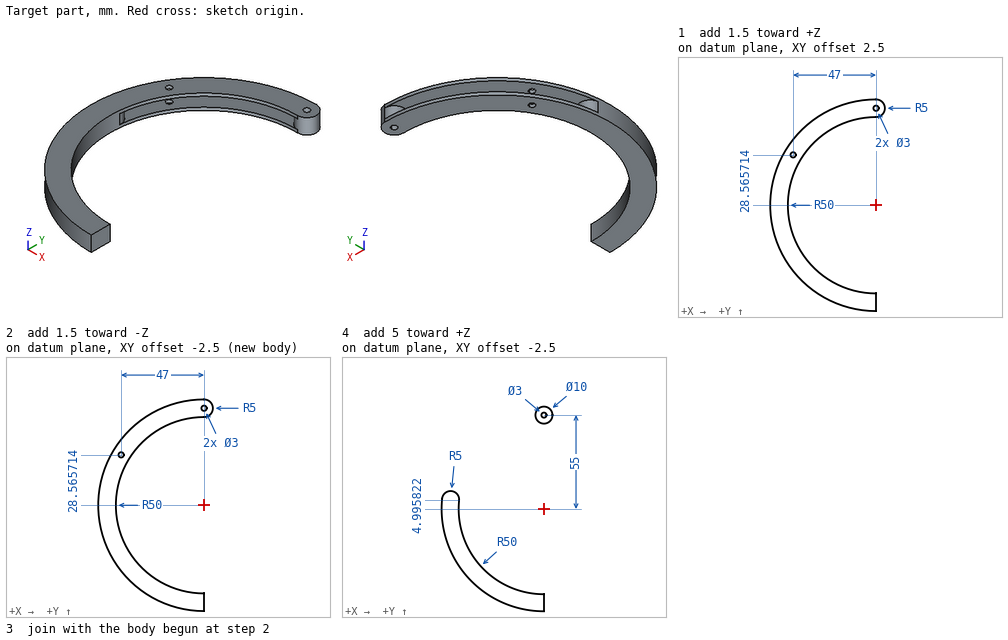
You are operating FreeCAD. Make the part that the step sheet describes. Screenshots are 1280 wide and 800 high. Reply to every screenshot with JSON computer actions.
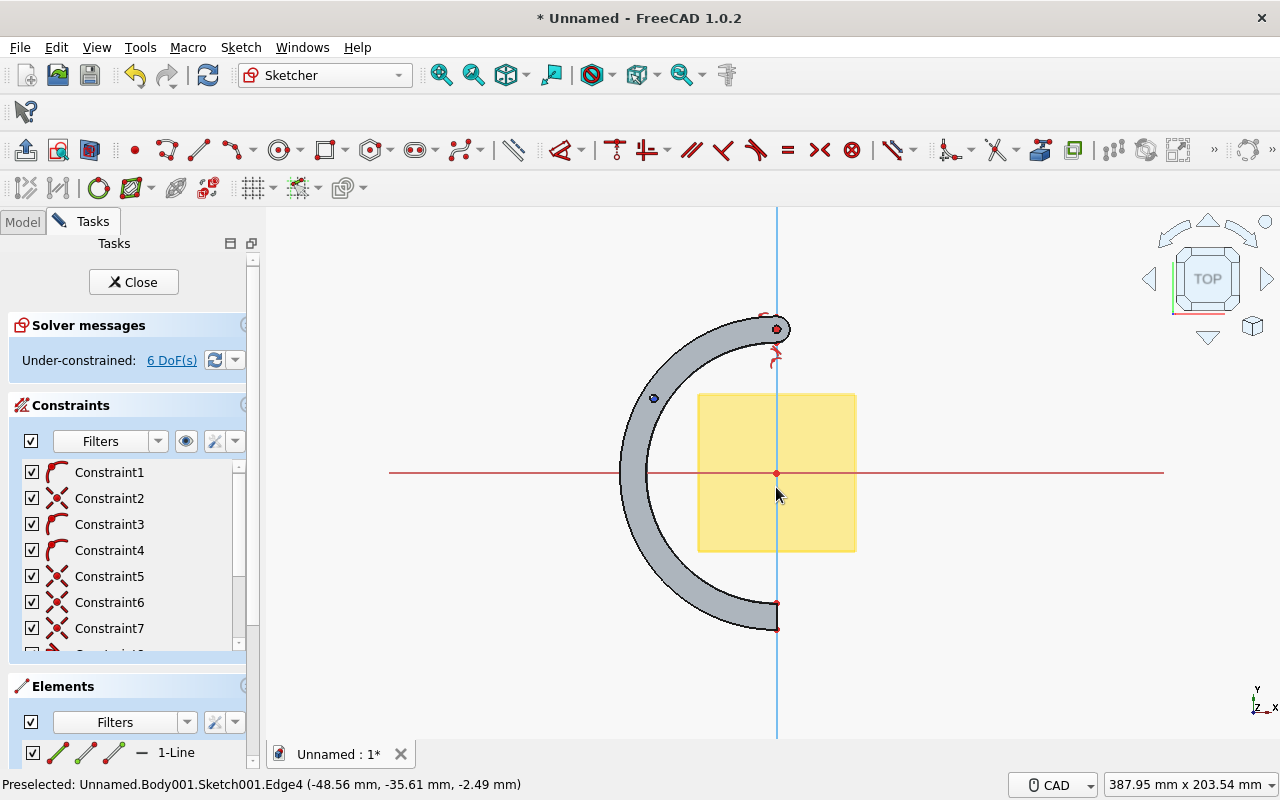
{"action": "scroll", "coordinate": [656, 398], "scroll_direction": "up", "scroll_amount": 8}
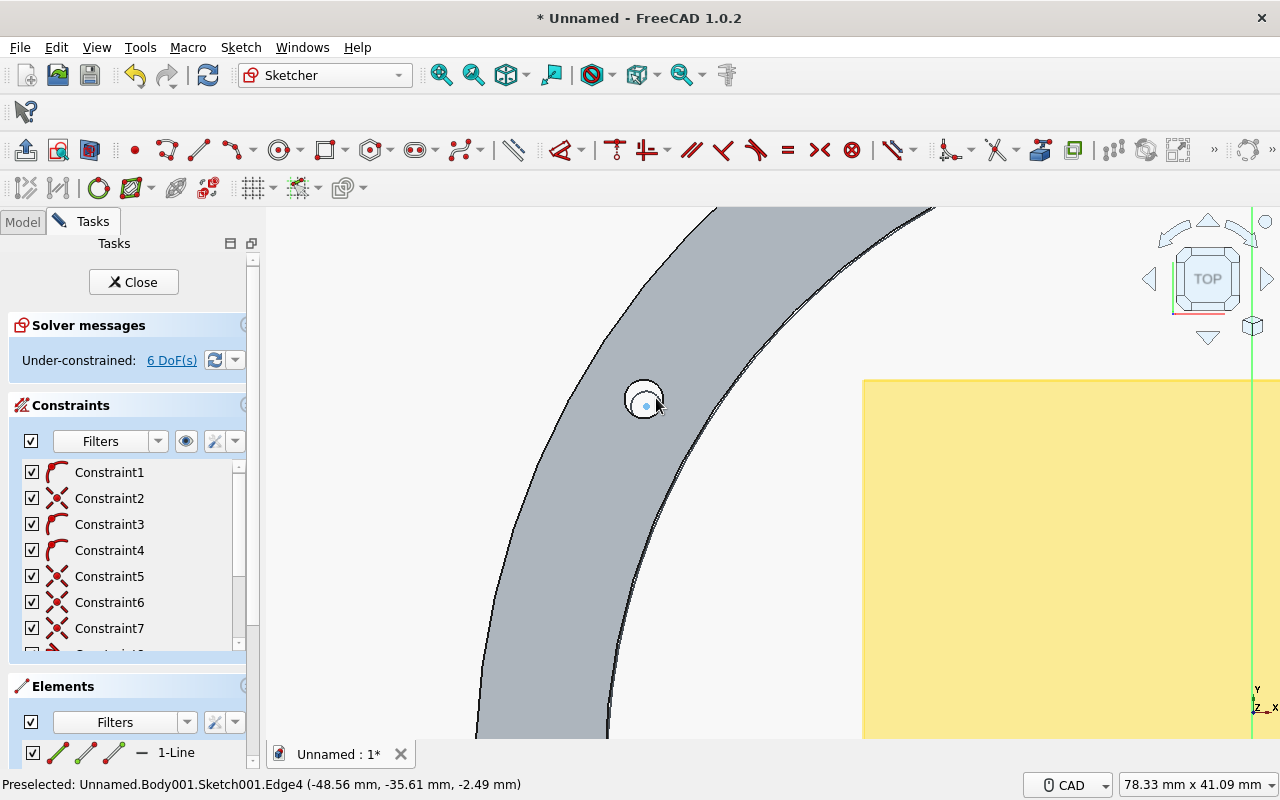
{"action": "left_click", "coordinate": [657, 396]}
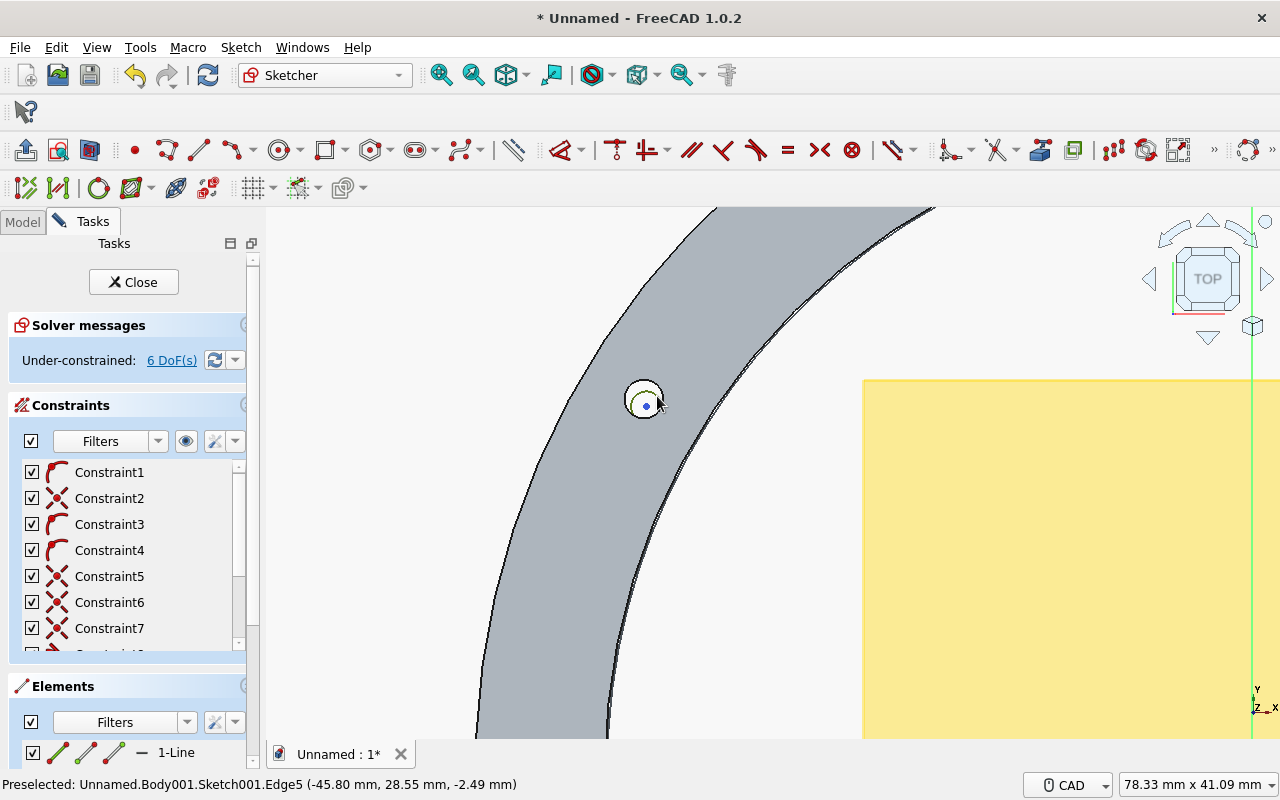
{"action": "scroll", "coordinate": [656, 398], "scroll_direction": "down", "scroll_amount": 8}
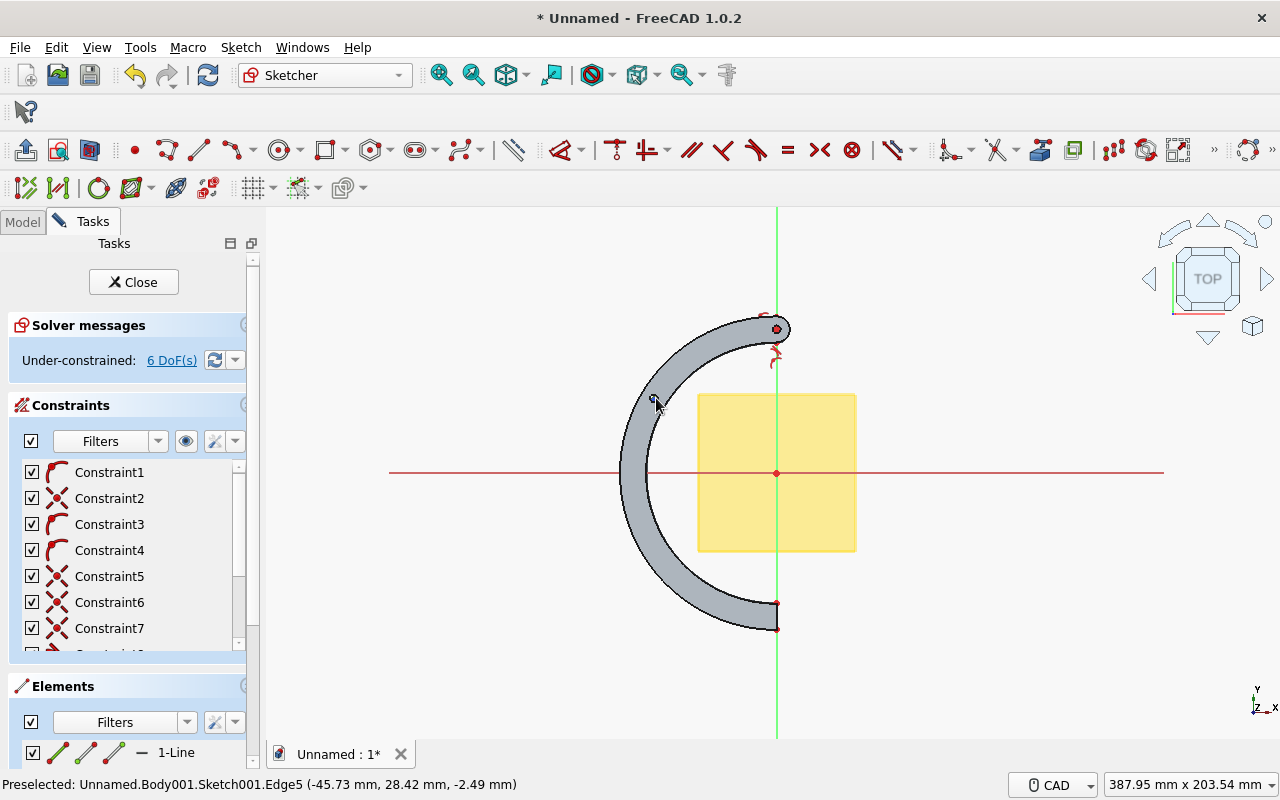
{"action": "scroll", "coordinate": [780, 327], "scroll_direction": "up", "scroll_amount": 8}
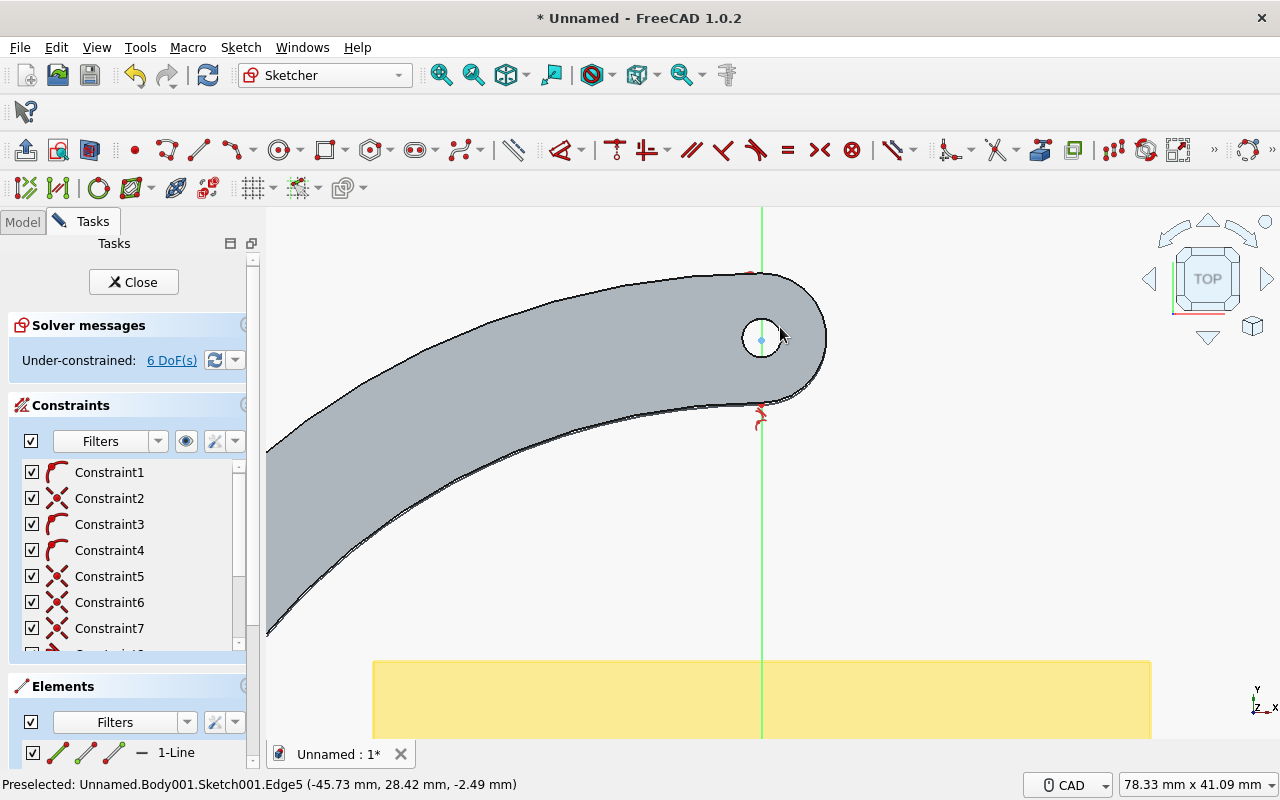
{"action": "left_click", "coordinate": [777, 325]}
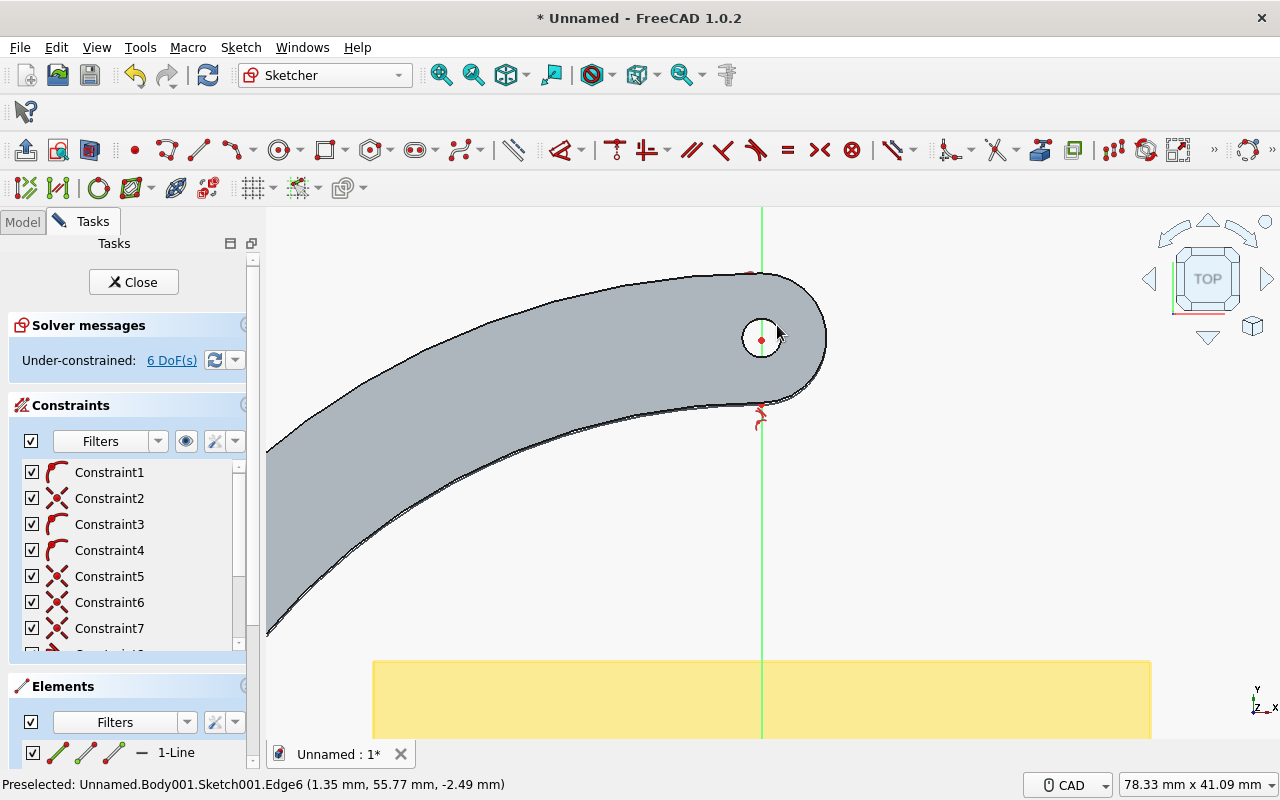
{"action": "left_click", "coordinate": [788, 150]}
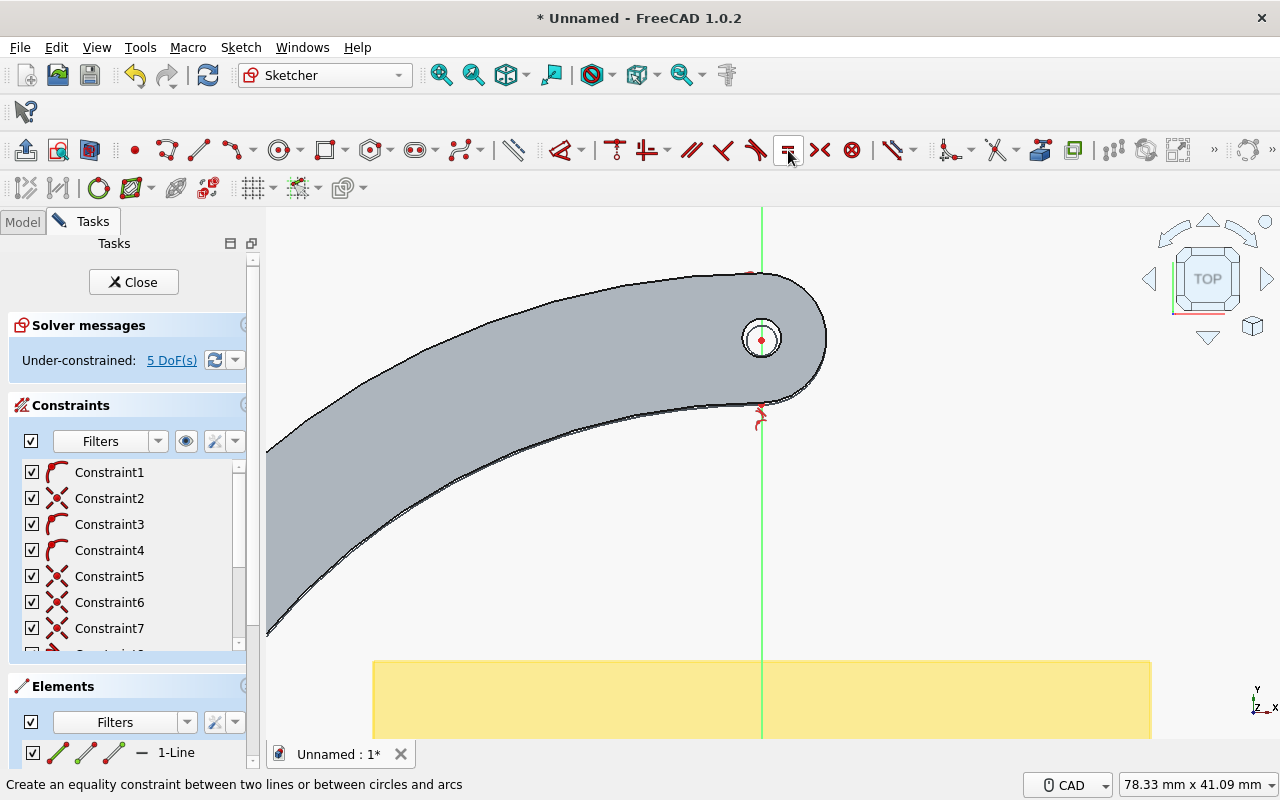
{"action": "left_click", "coordinate": [560, 150]}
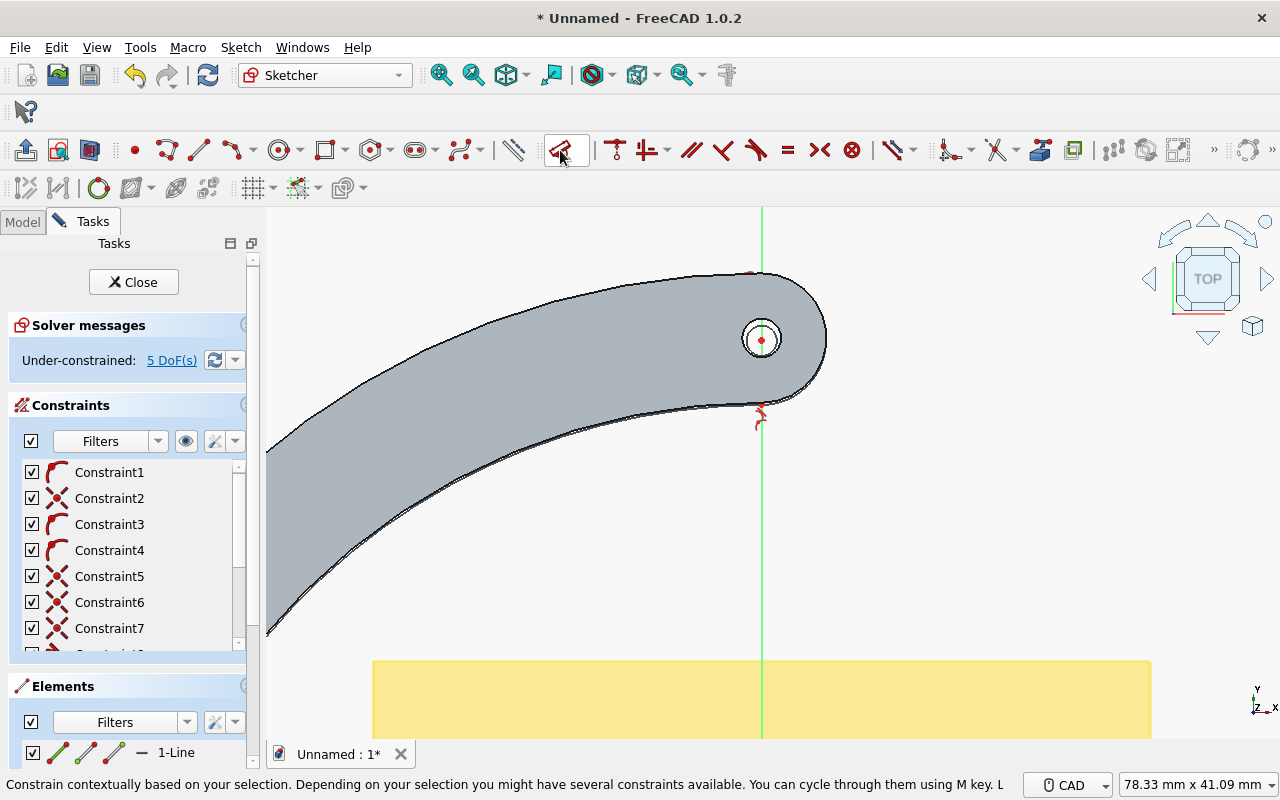
{"action": "scroll", "coordinate": [780, 327], "scroll_direction": "down", "scroll_amount": 8}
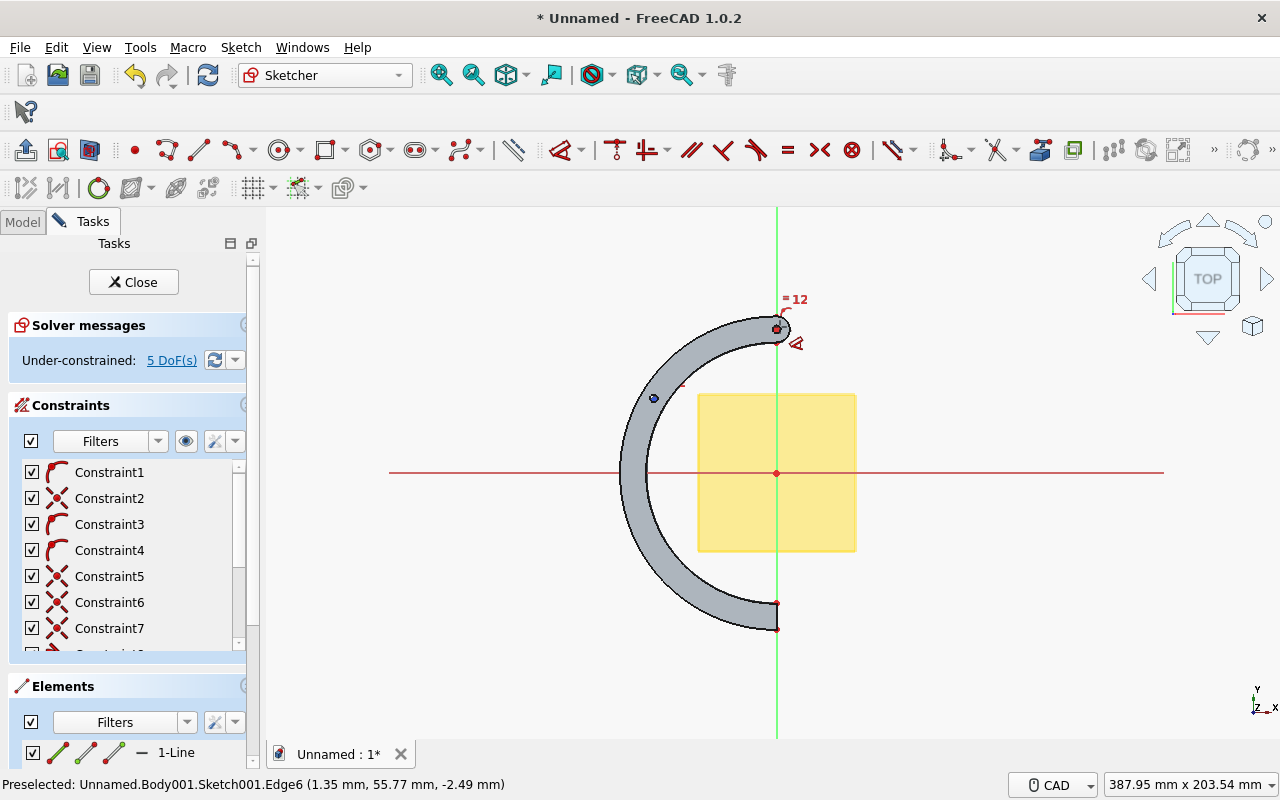
{"action": "left_click", "coordinate": [700, 368]}
{"action": "left_click", "coordinate": [835, 322]}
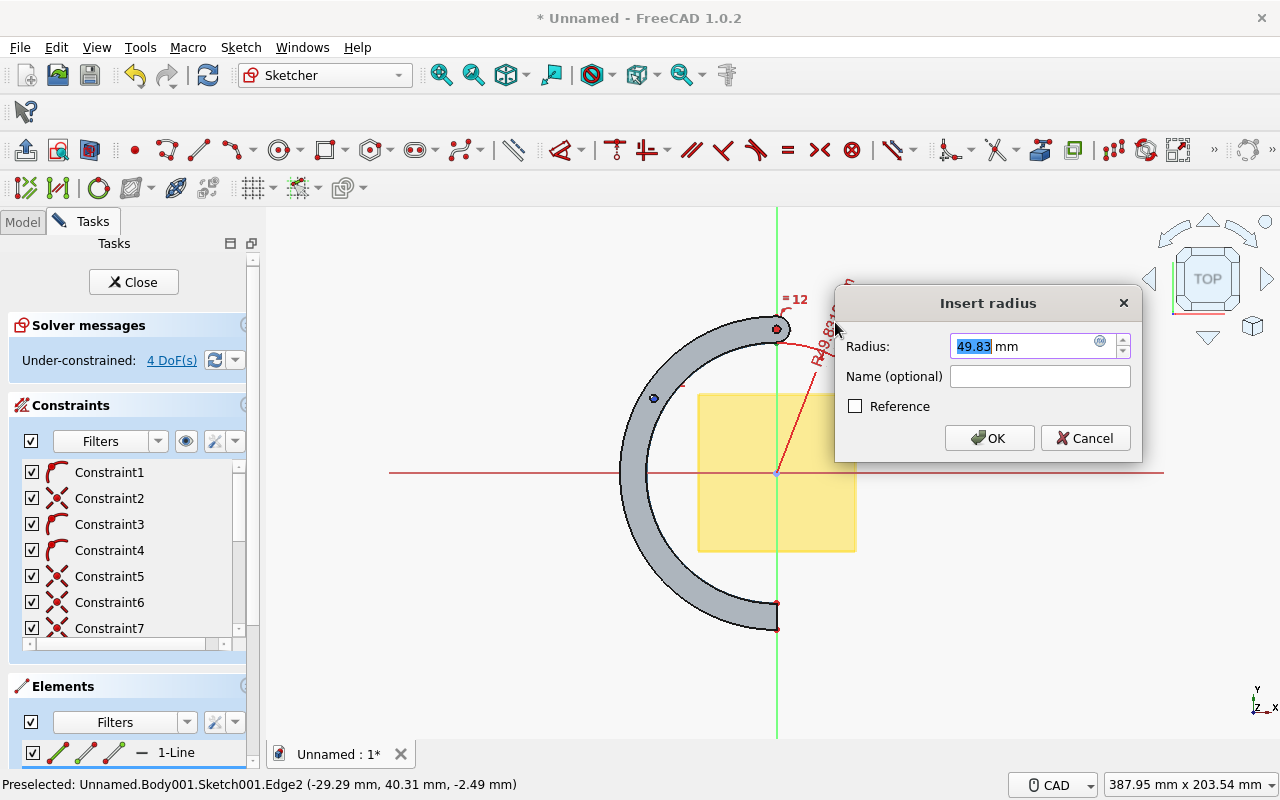
{"action": "type", "text": "50"}
{"action": "key", "text": "Return"}